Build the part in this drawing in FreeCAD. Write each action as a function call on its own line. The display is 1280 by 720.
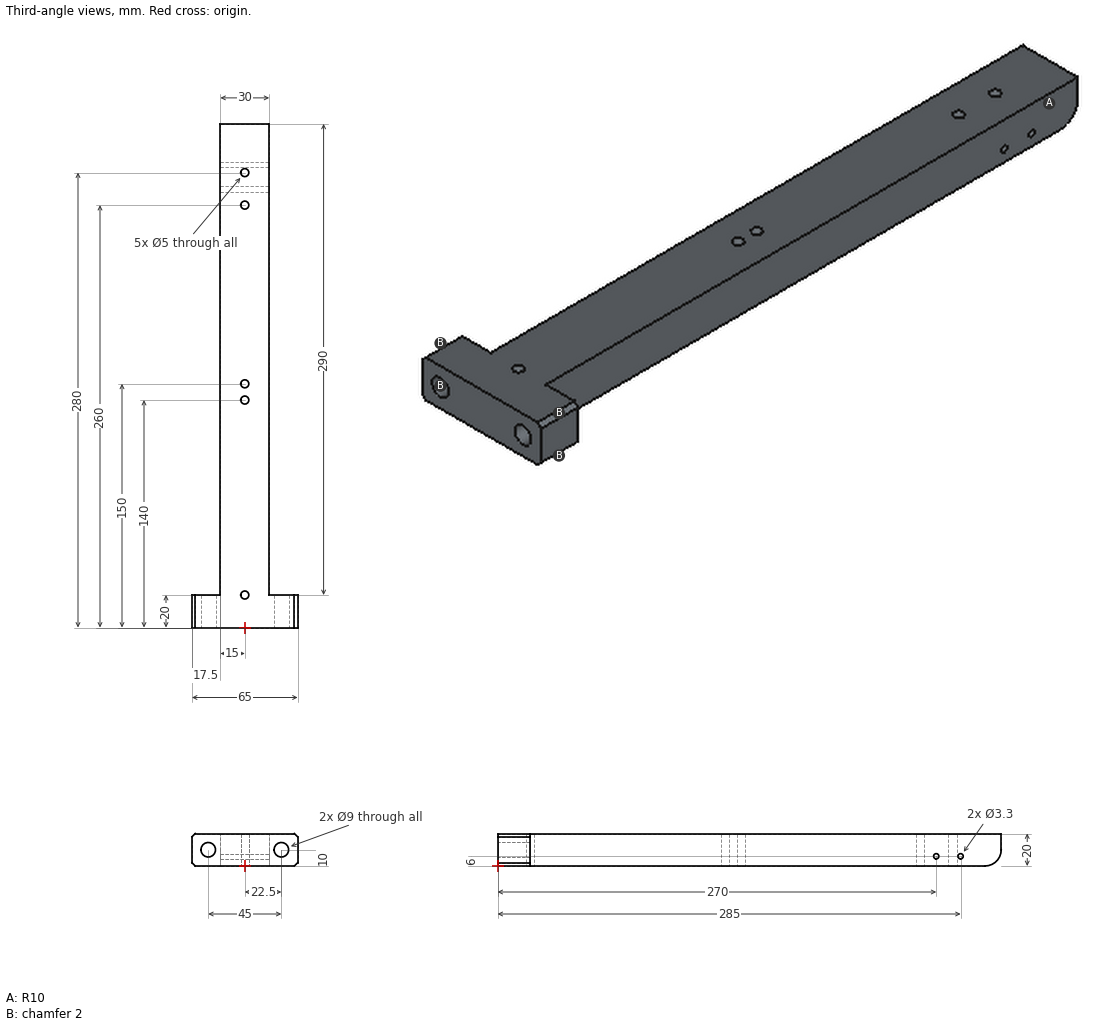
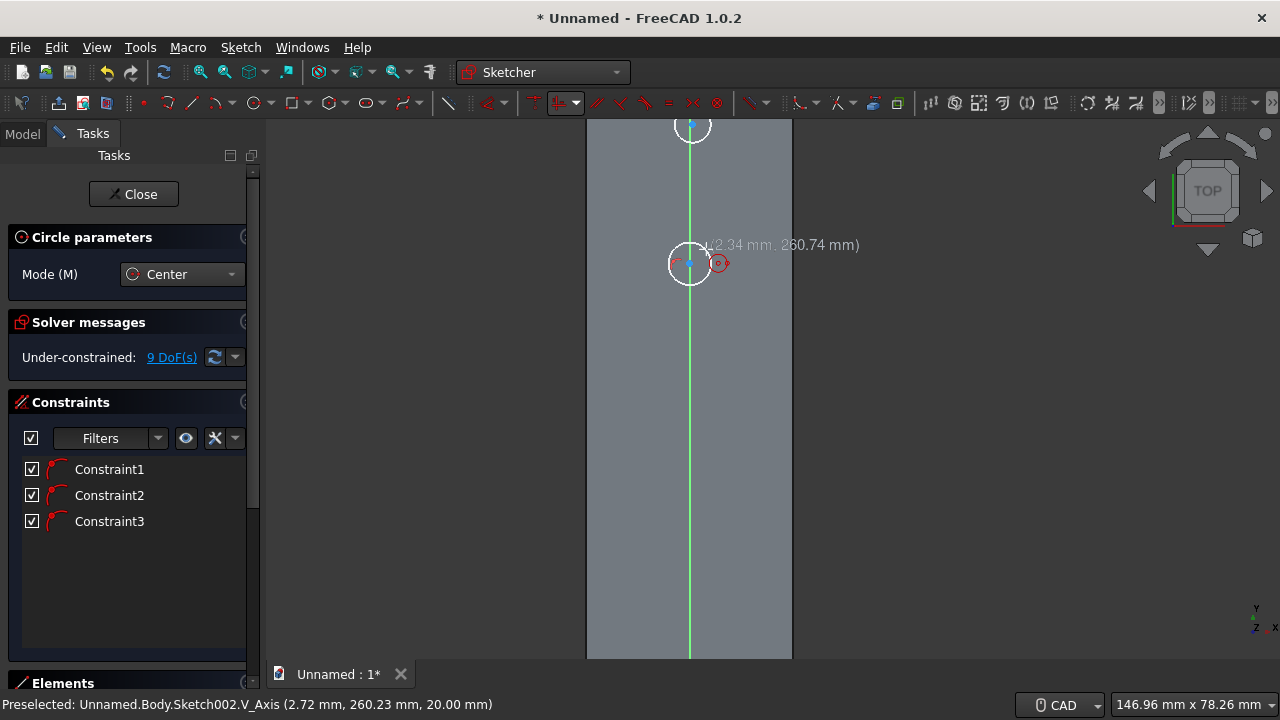
scroll(707, 253, down, 9)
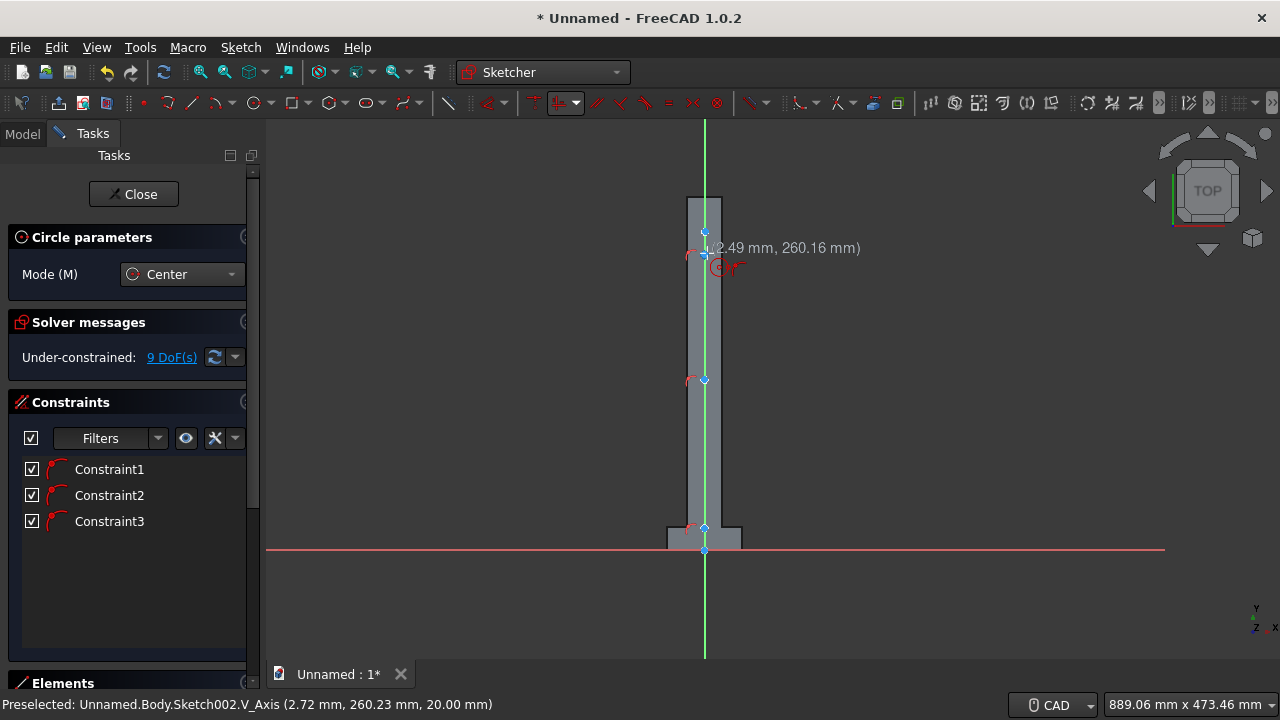
scroll(705, 390, up, 11)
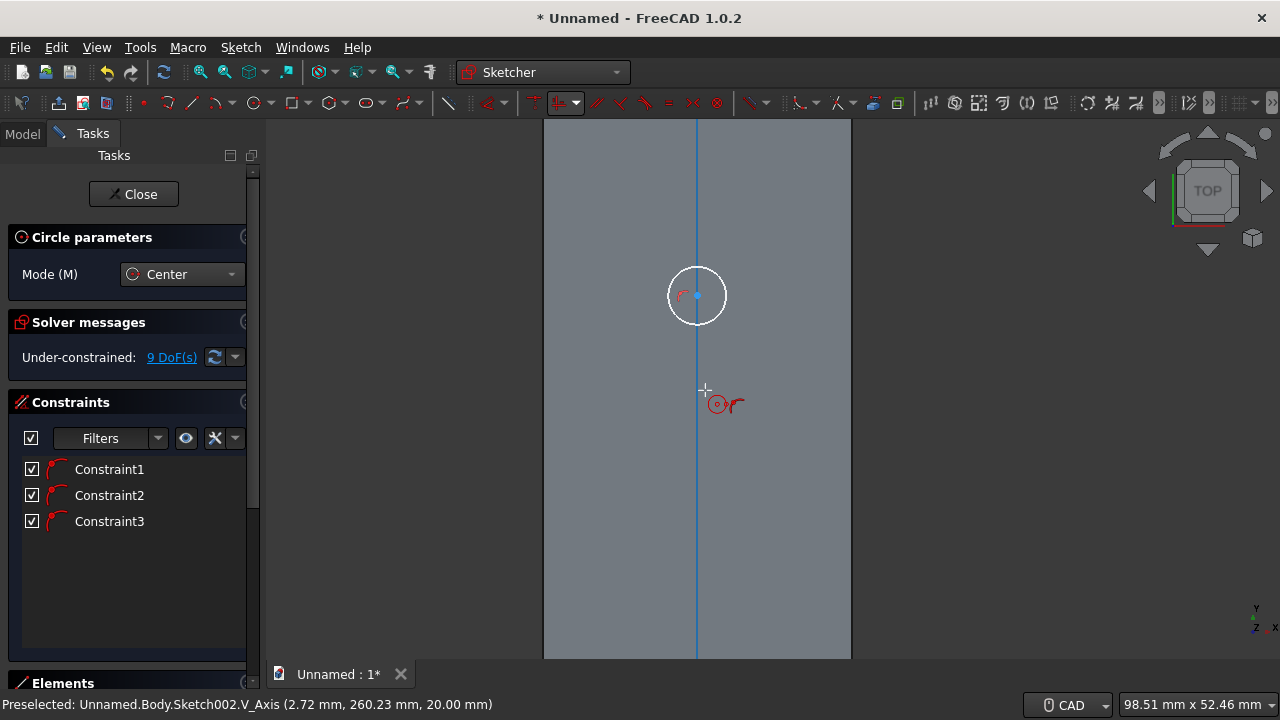
scroll(705, 391, down, 11)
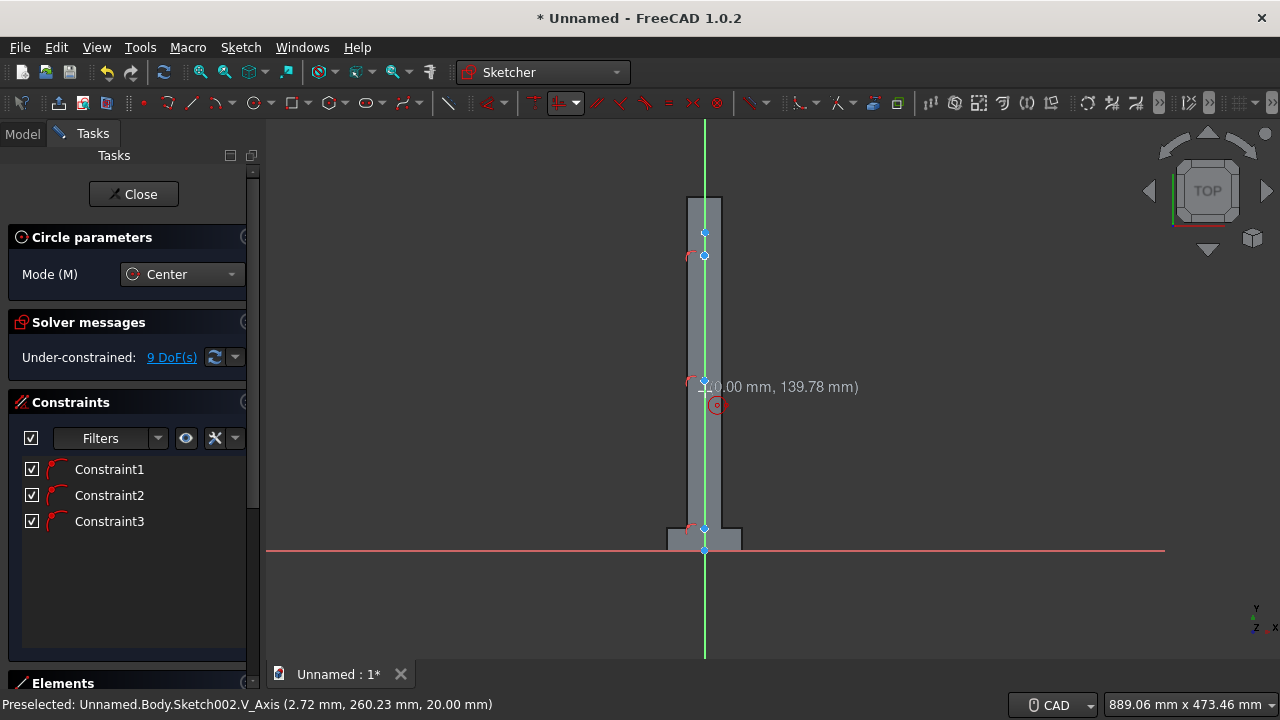
scroll(705, 391, up, 4)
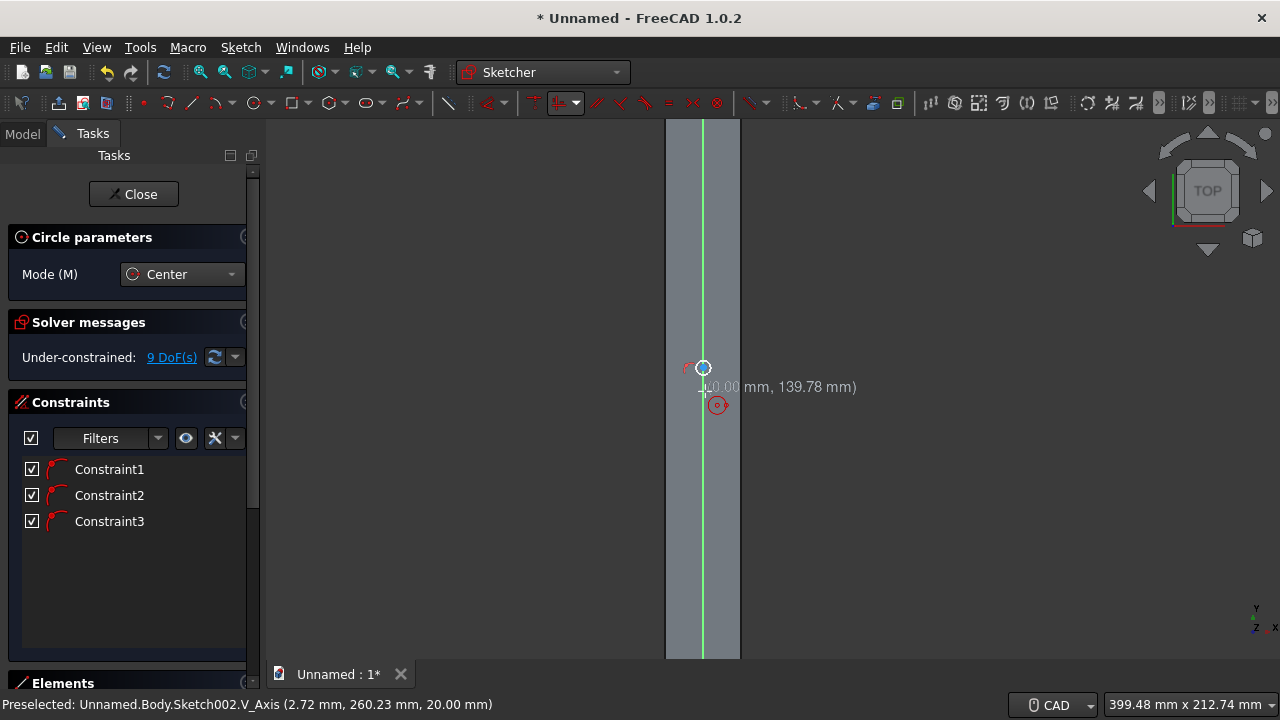
click(703, 391)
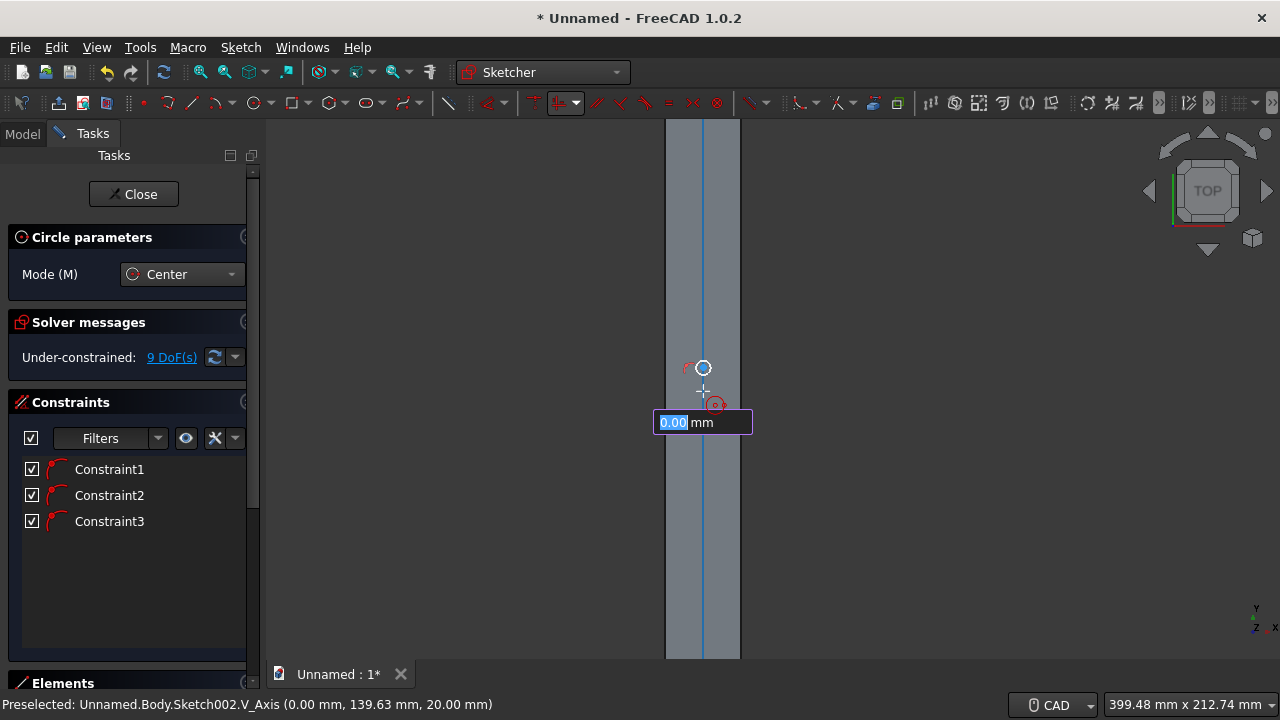
scroll(709, 389, up, 5)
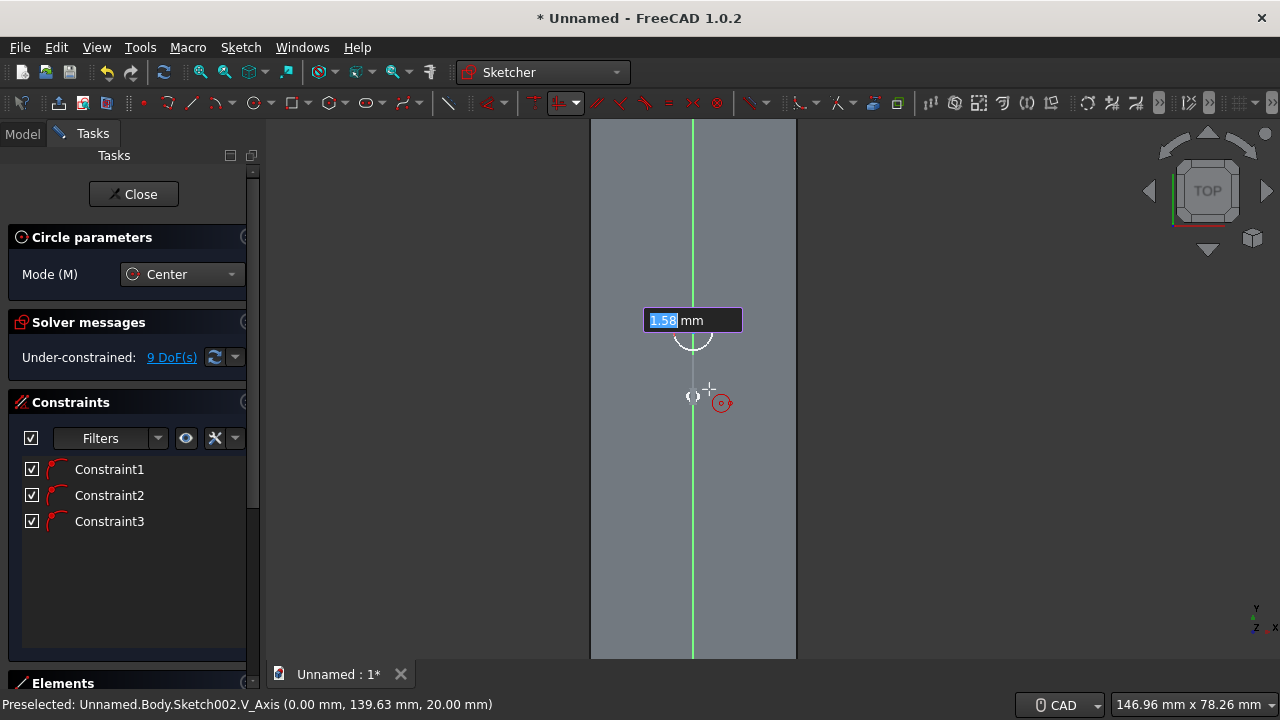
click(709, 388)
key(Escape)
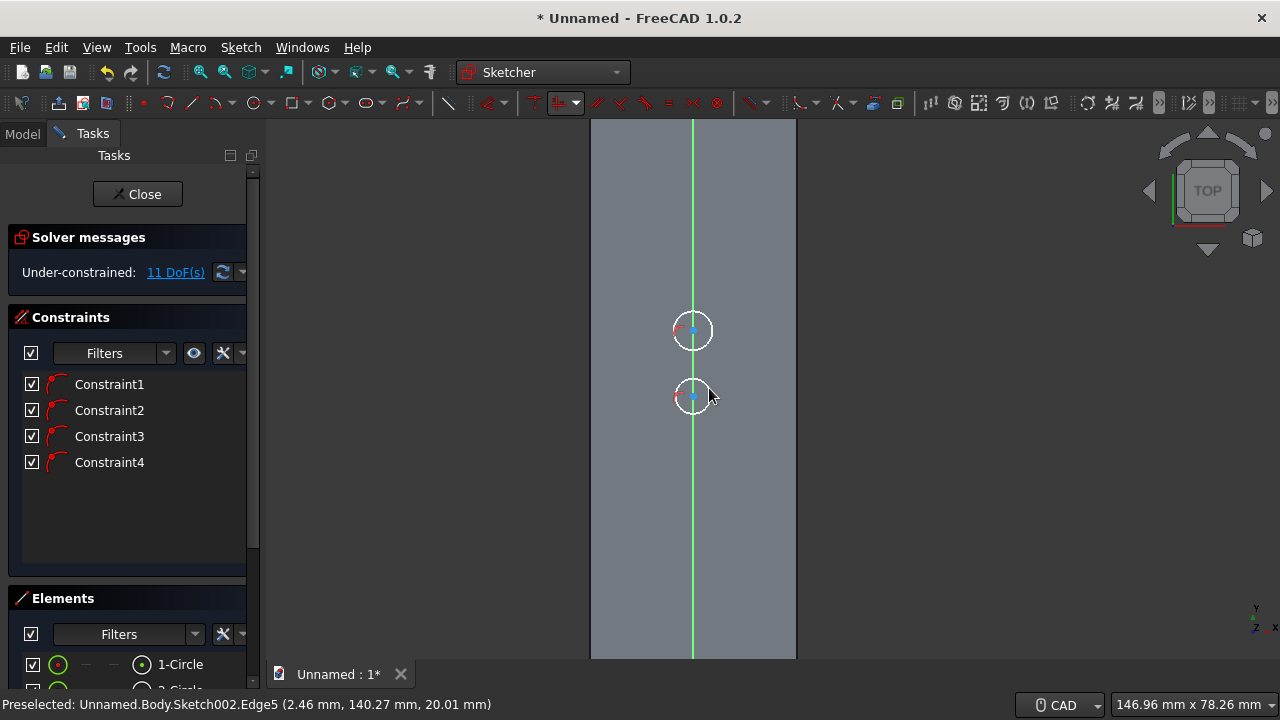
scroll(707, 390, down, 9)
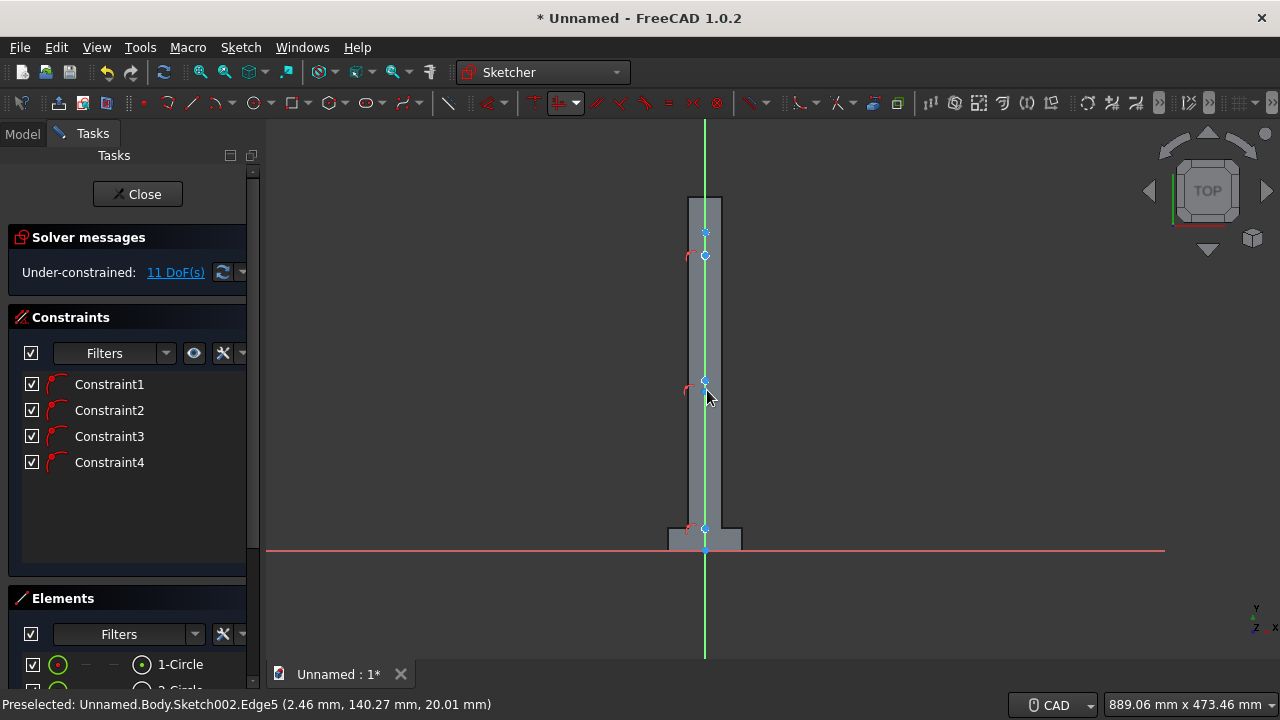
scroll(708, 231, up, 9)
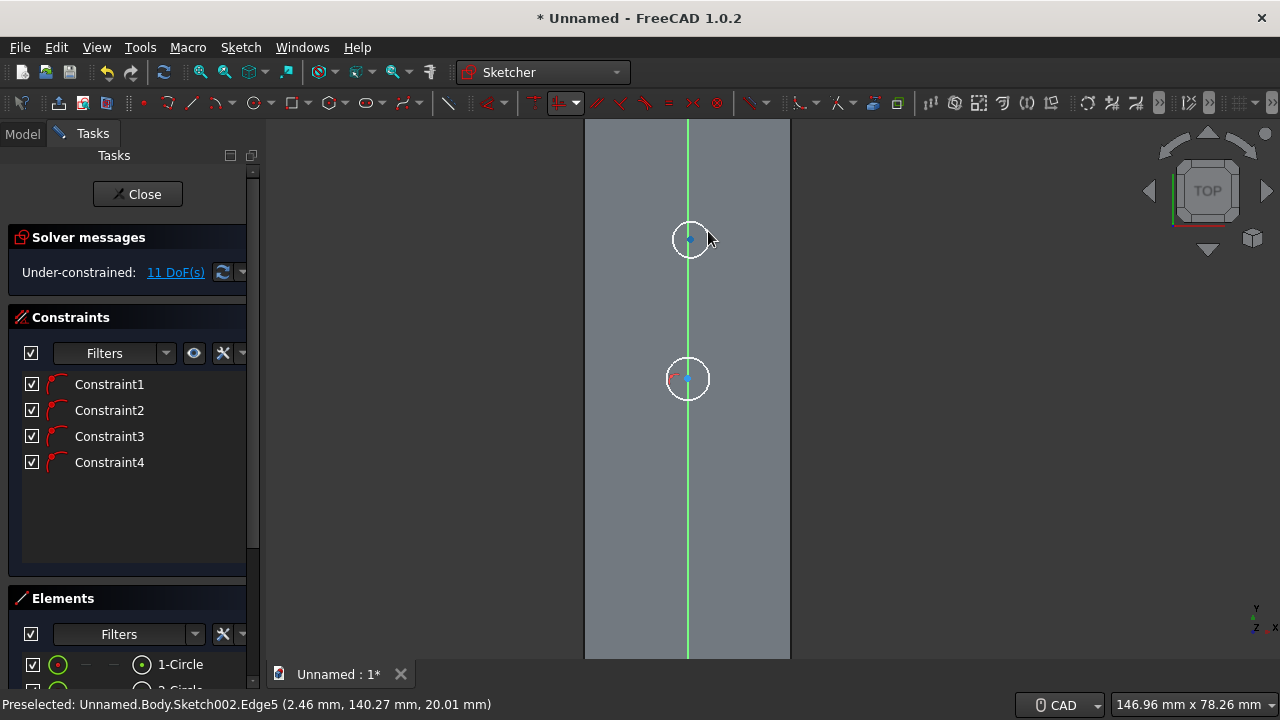
click(704, 227)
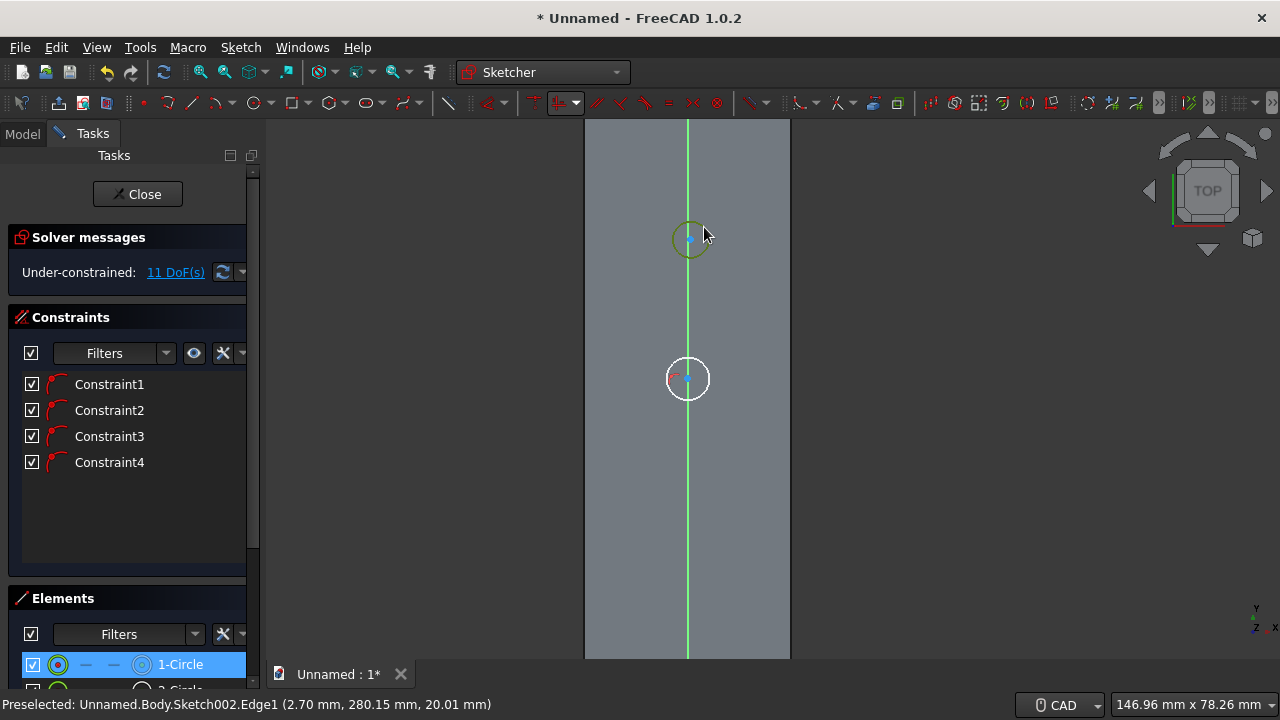
scroll(708, 230, down, 9)